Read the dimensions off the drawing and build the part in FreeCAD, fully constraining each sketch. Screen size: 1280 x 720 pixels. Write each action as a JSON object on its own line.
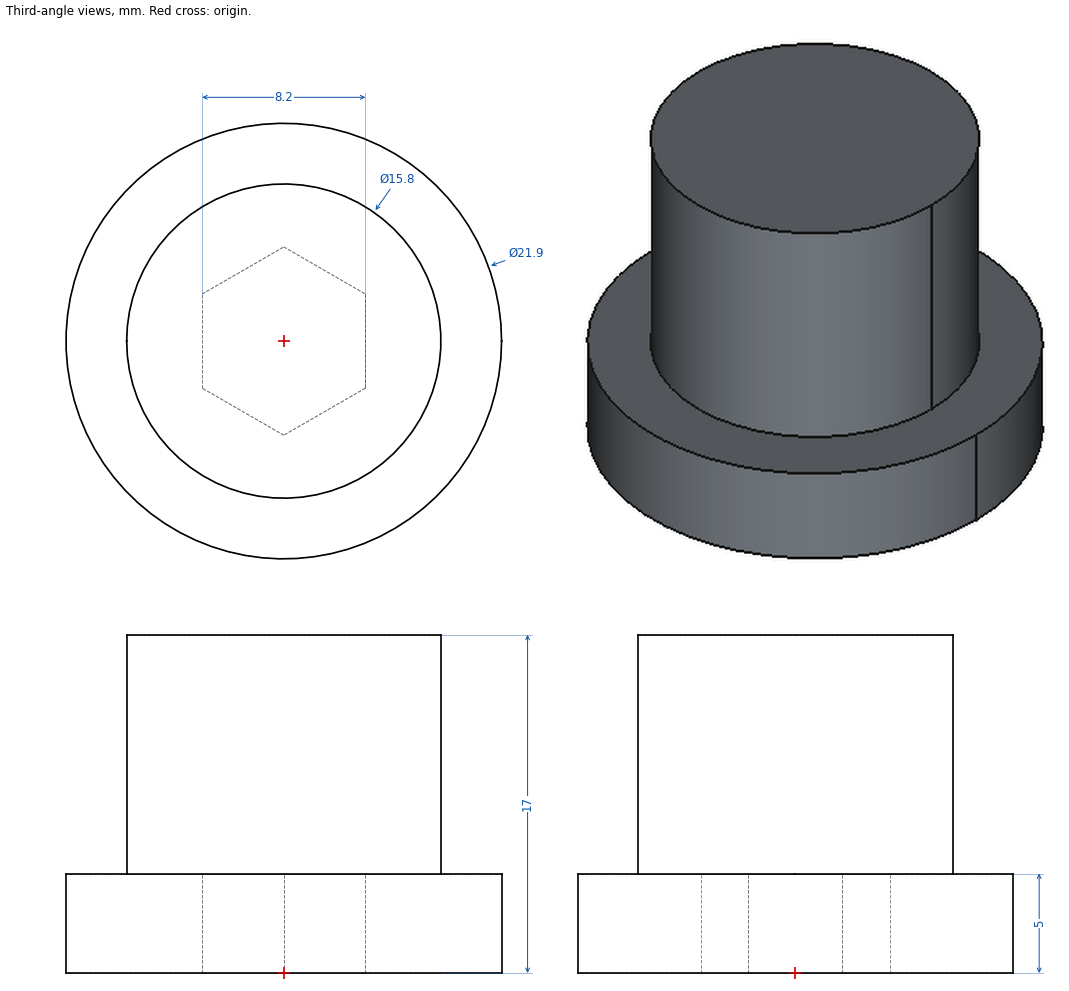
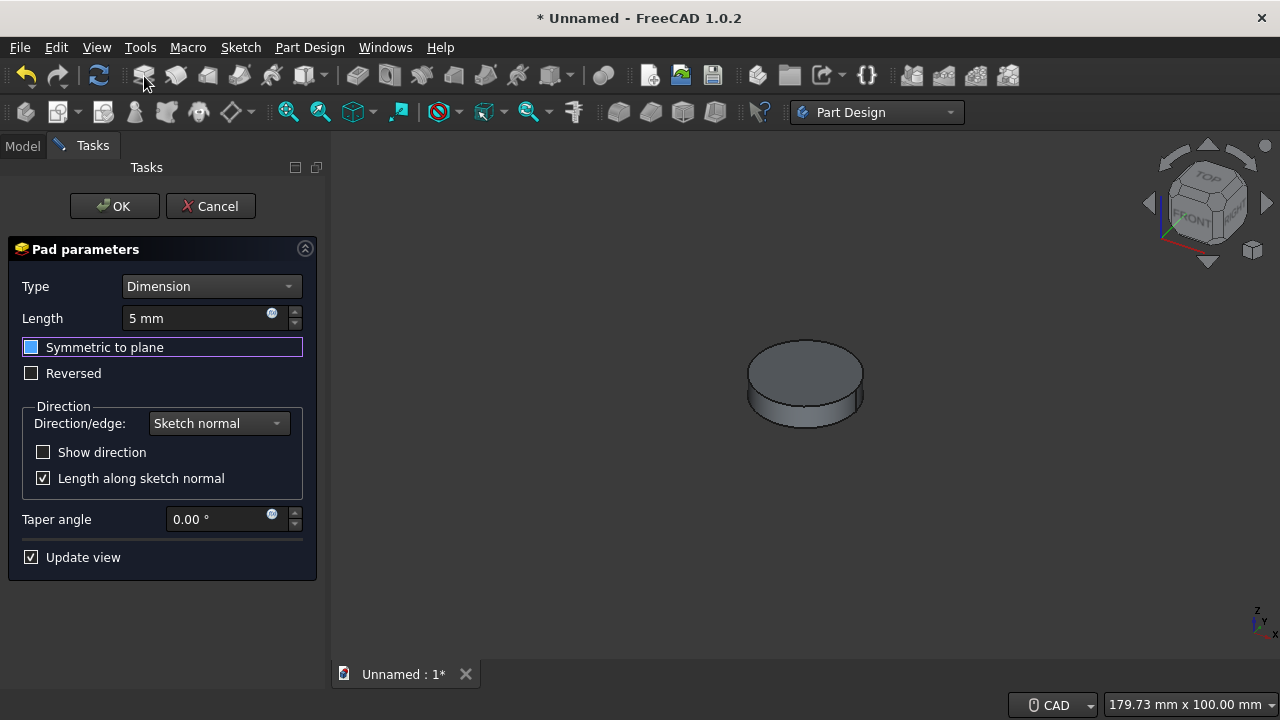
{"action": "left_click", "coordinate": [115, 206]}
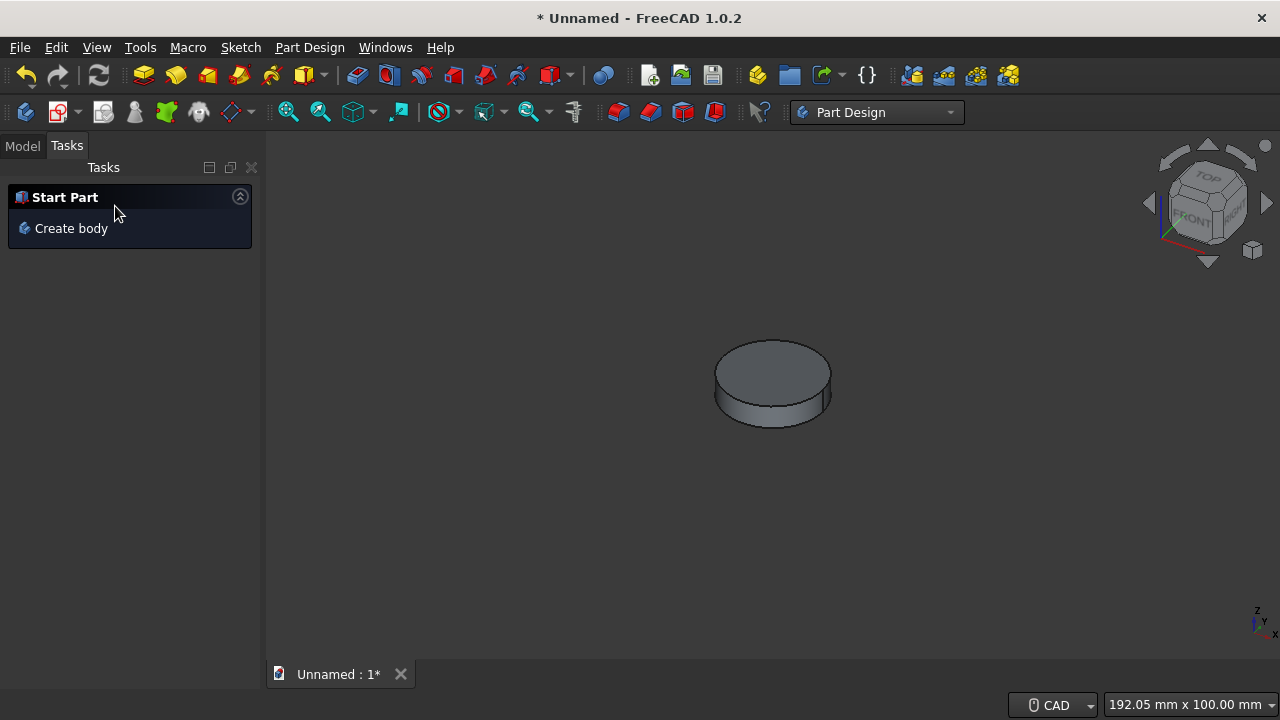
{"action": "key", "text": "v f"}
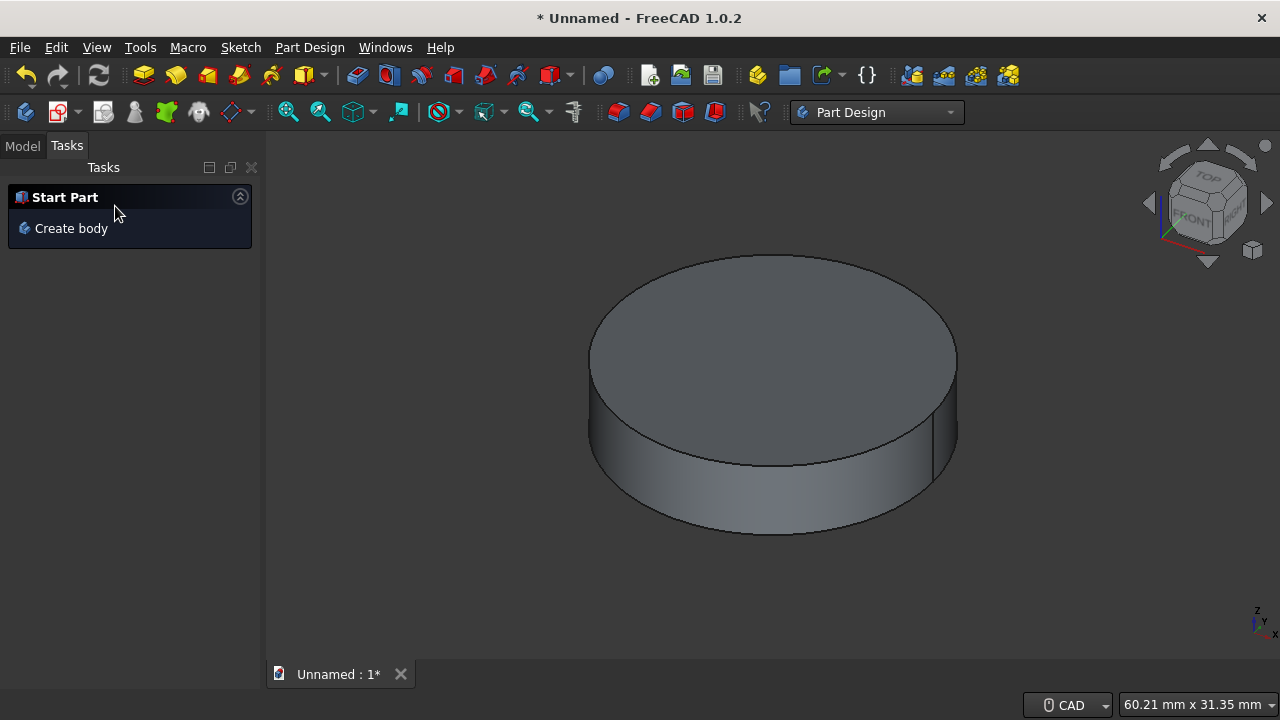
{"action": "key", "text": "5"}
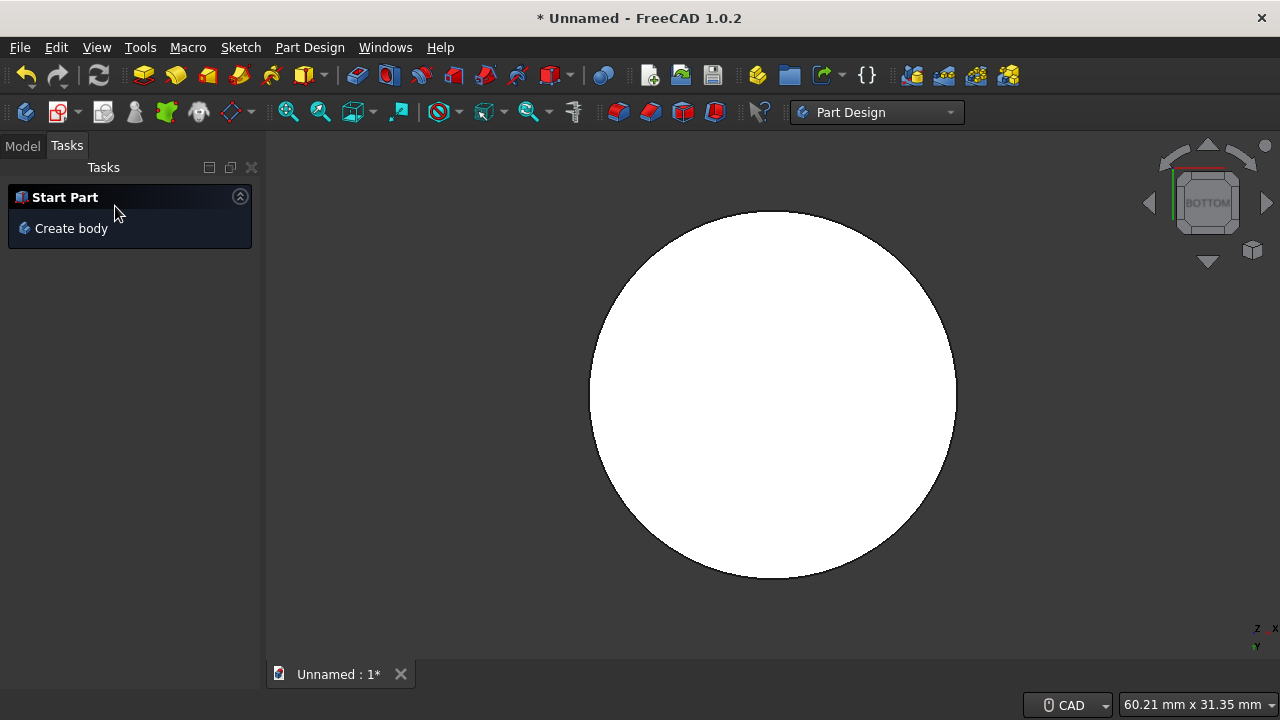
{"action": "left_click", "coordinate": [773, 394]}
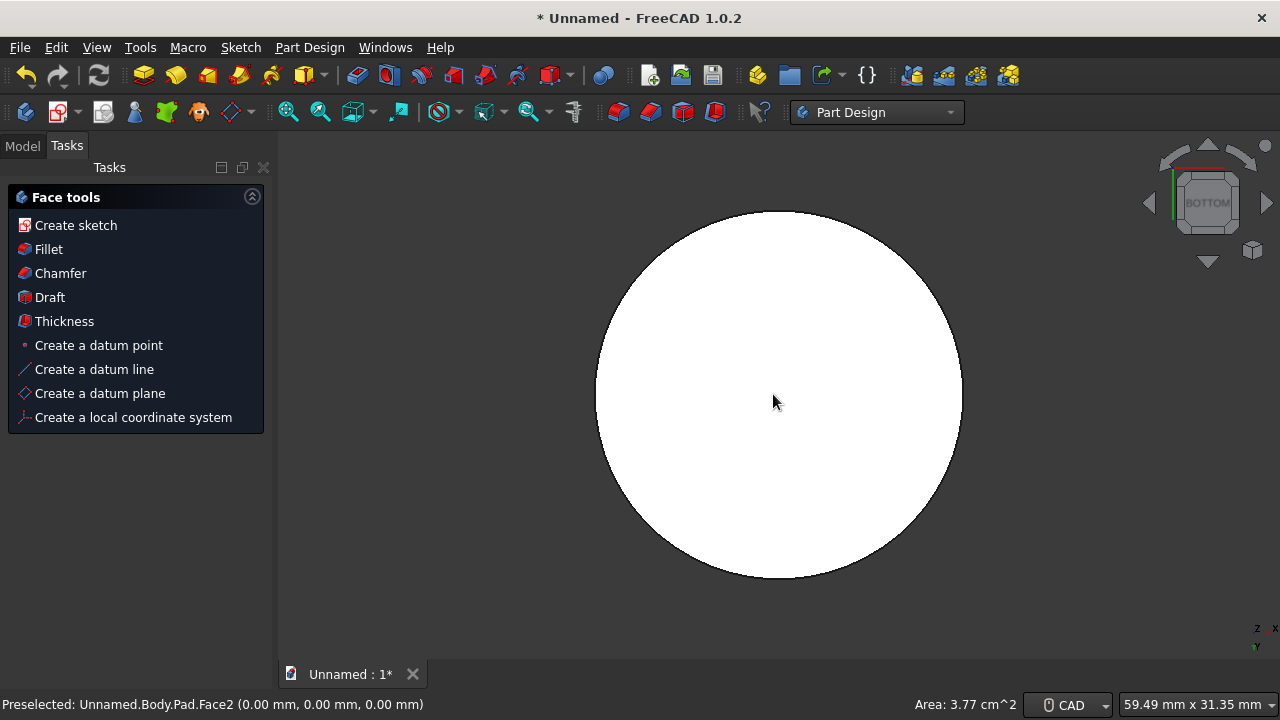
{"action": "left_click", "coordinate": [58, 112]}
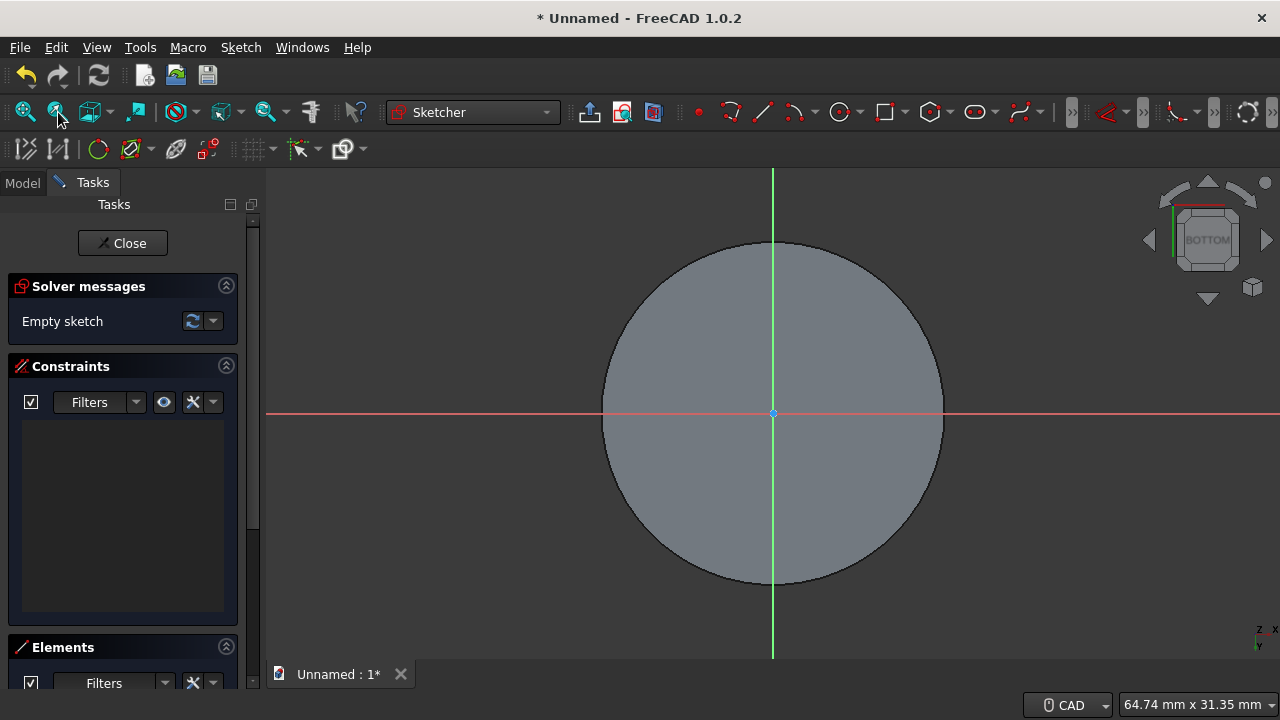
{"action": "key", "text": "g c"}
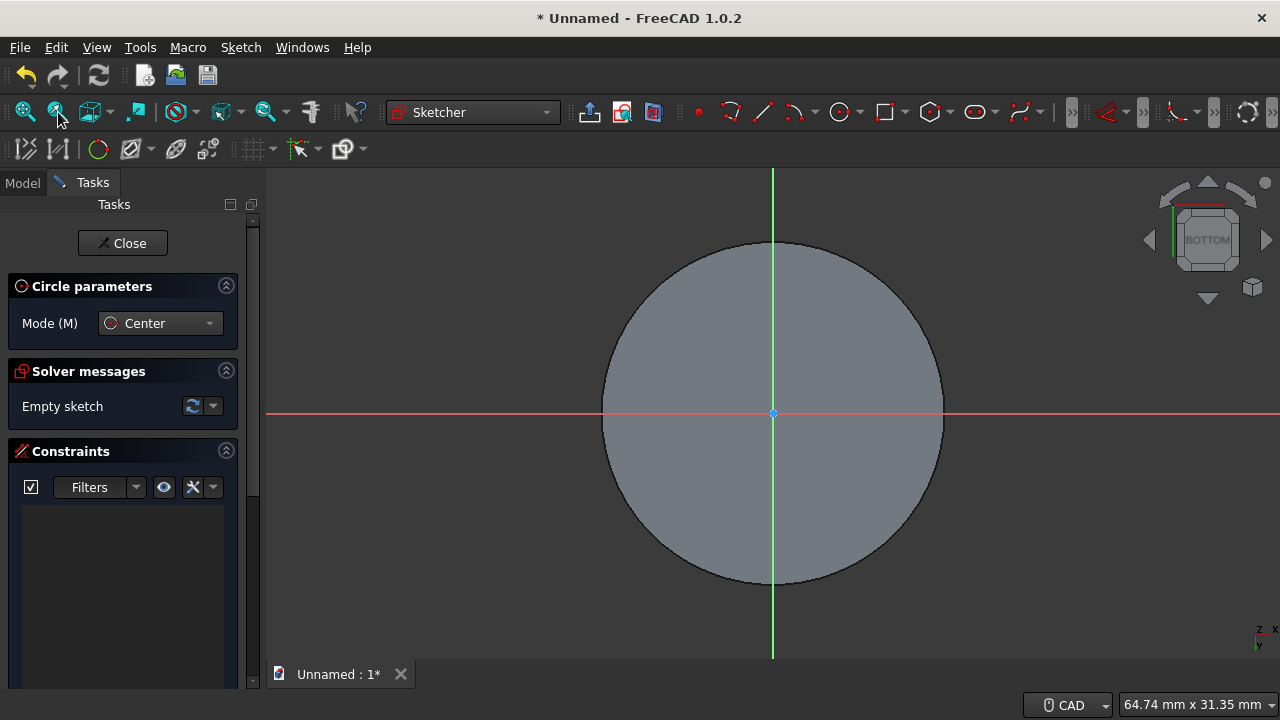
{"action": "left_click", "coordinate": [773, 414]}
{"action": "mouse_move", "coordinate": [860, 326]}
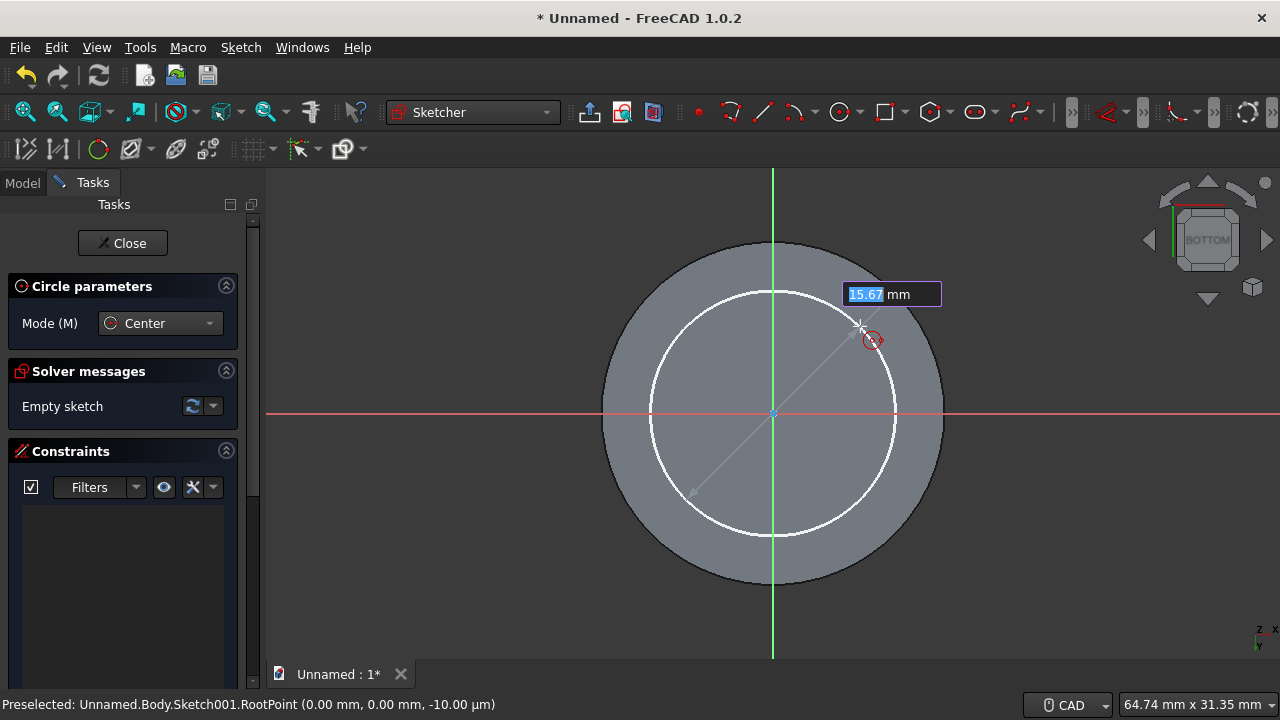
{"action": "type", "text": "15.8"}
{"action": "key", "text": "Return"}
{"action": "key", "text": "Escape"}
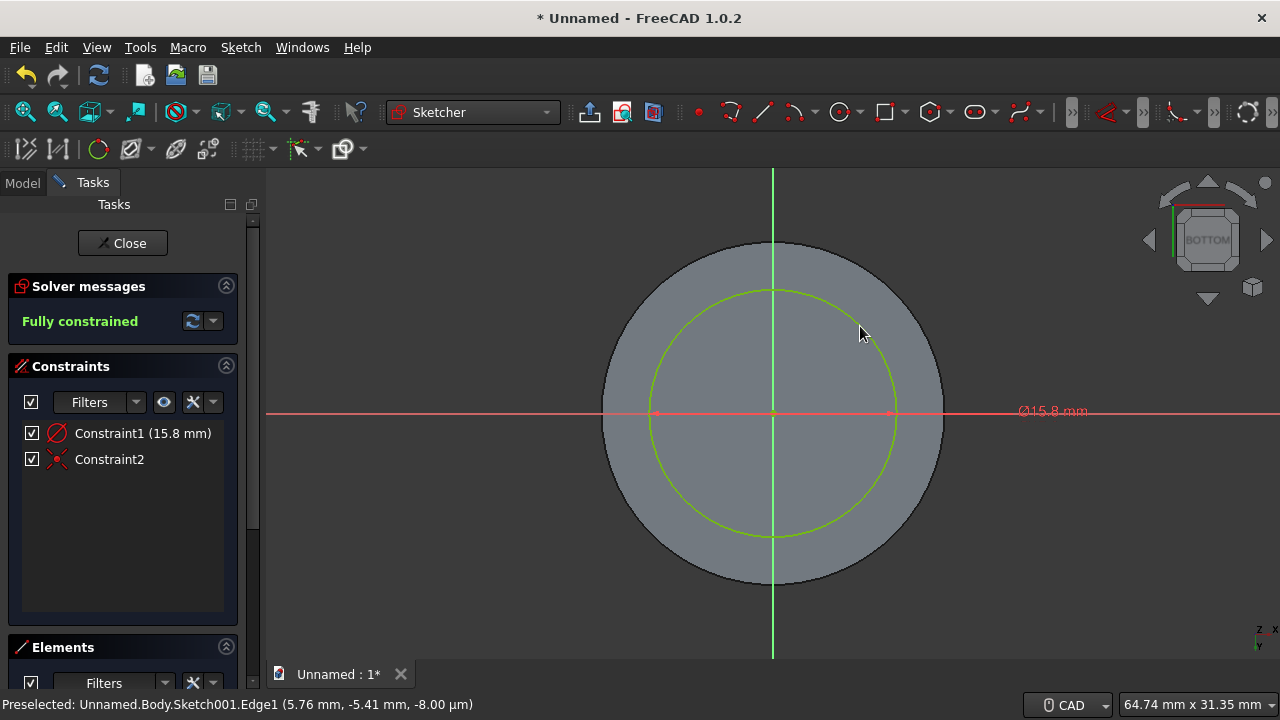
{"action": "left_click", "coordinate": [123, 243]}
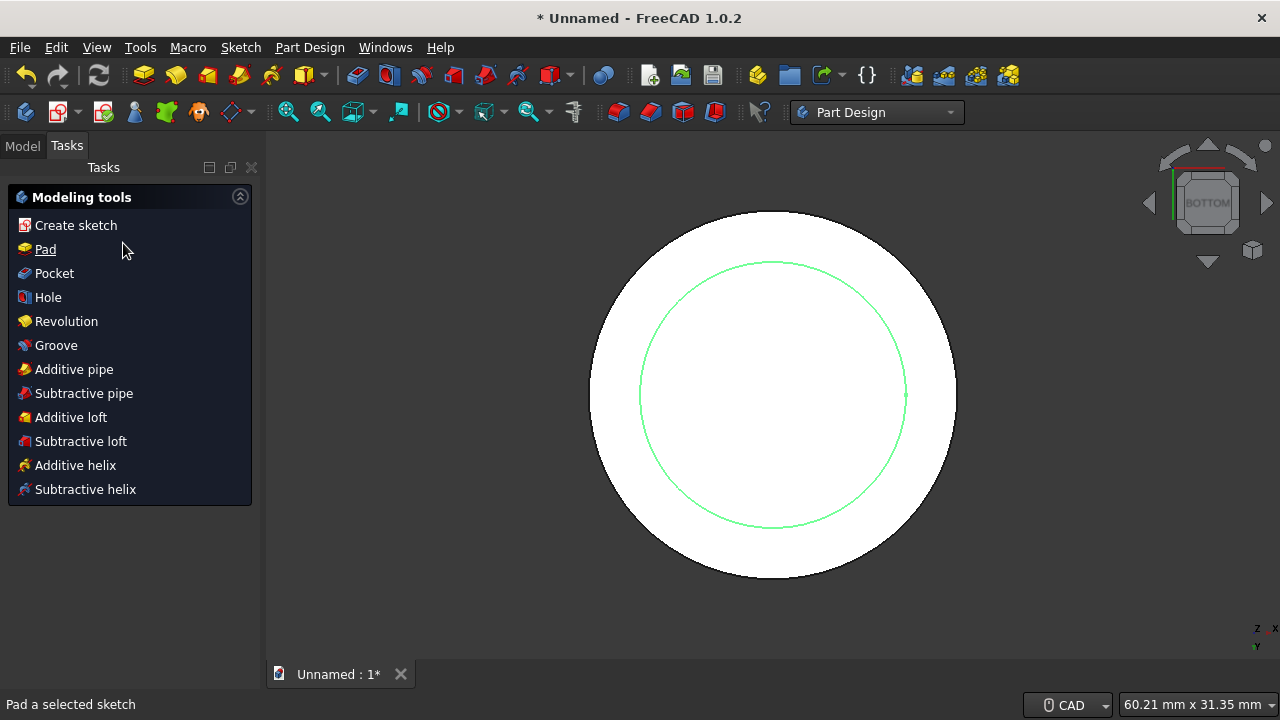
{"action": "left_click", "coordinate": [144, 76]}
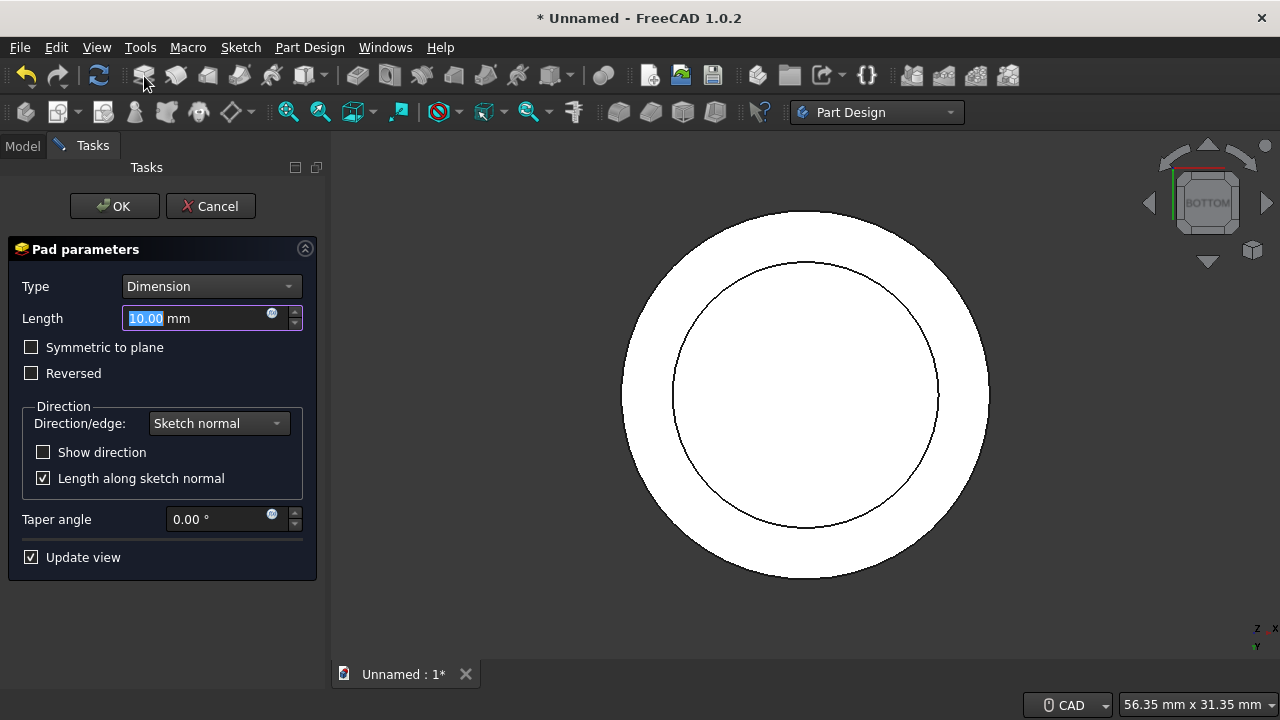
{"action": "type", "text": "17"}
{"action": "key", "text": "Tab"}